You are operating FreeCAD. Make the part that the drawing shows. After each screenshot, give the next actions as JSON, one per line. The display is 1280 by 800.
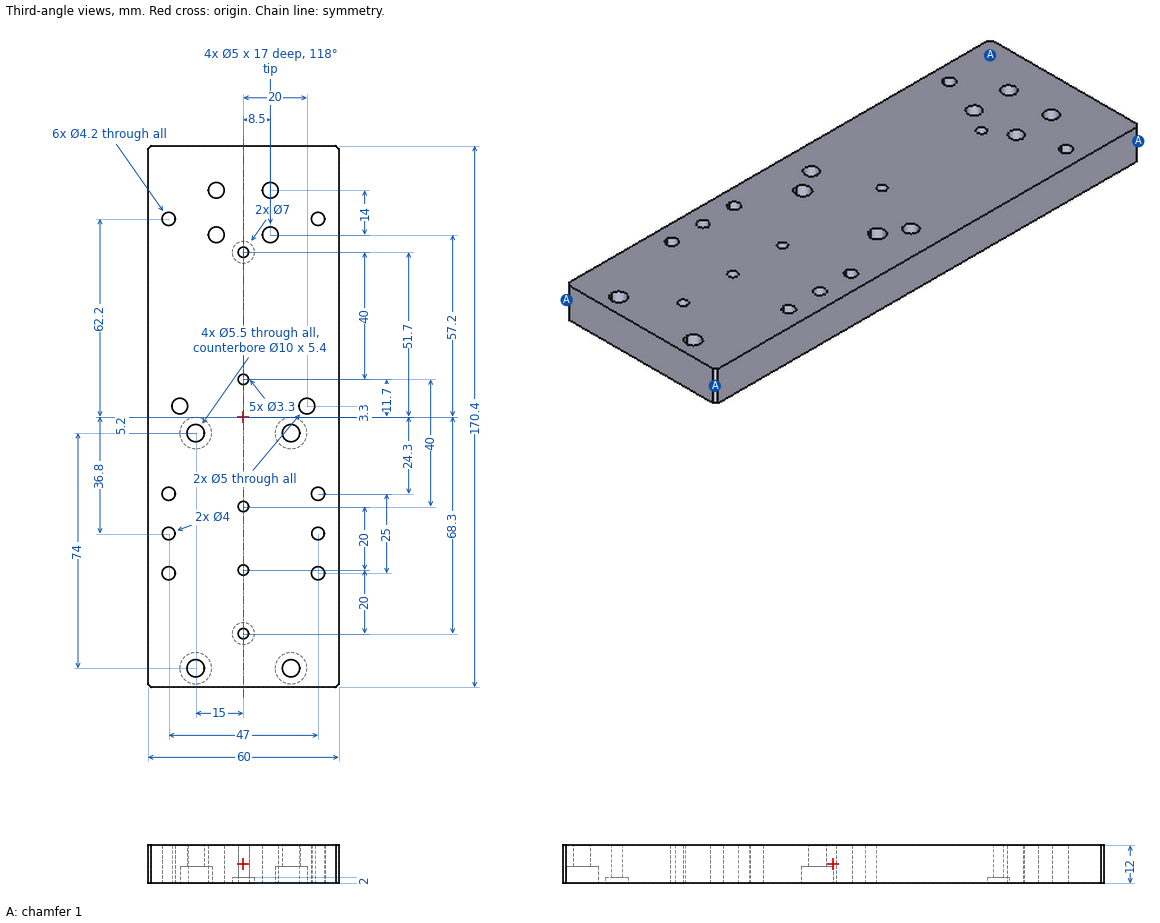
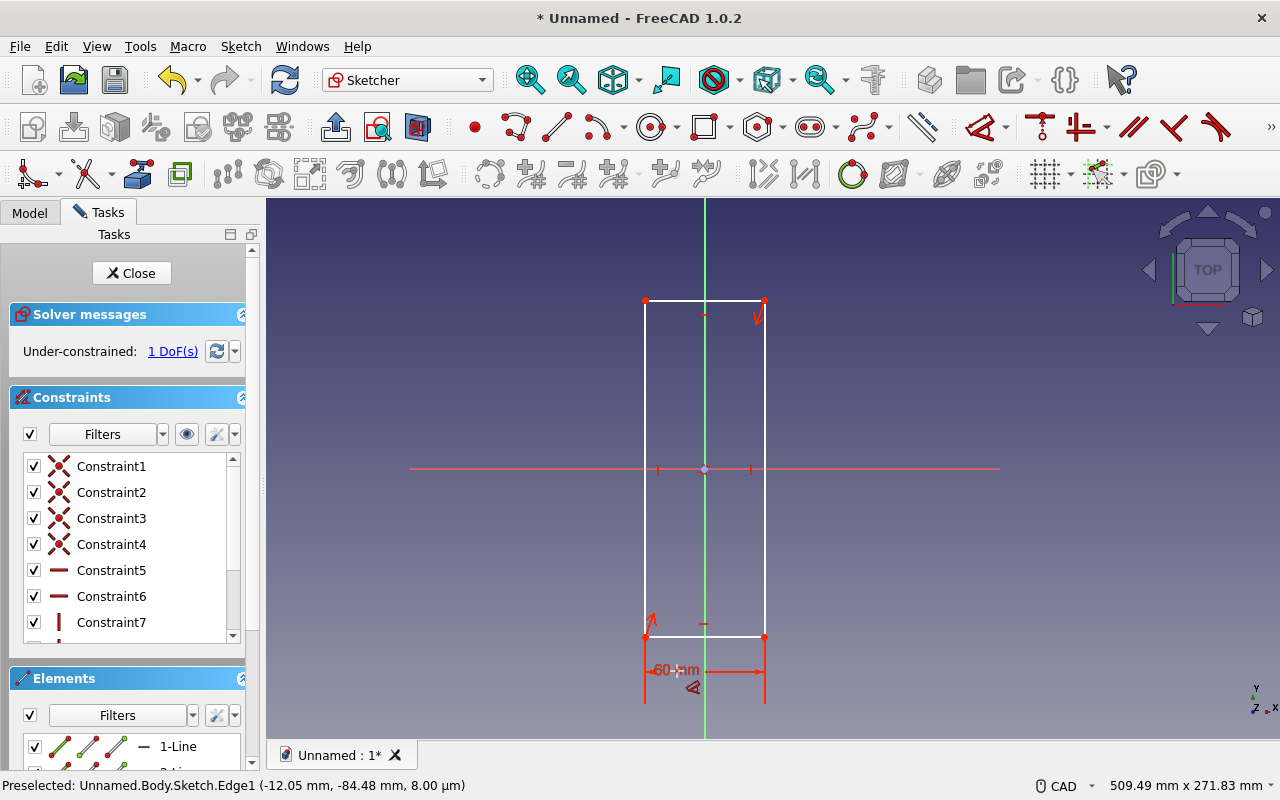
{"action": "left_click", "coordinate": [765, 536]}
{"action": "left_click", "coordinate": [799, 392]}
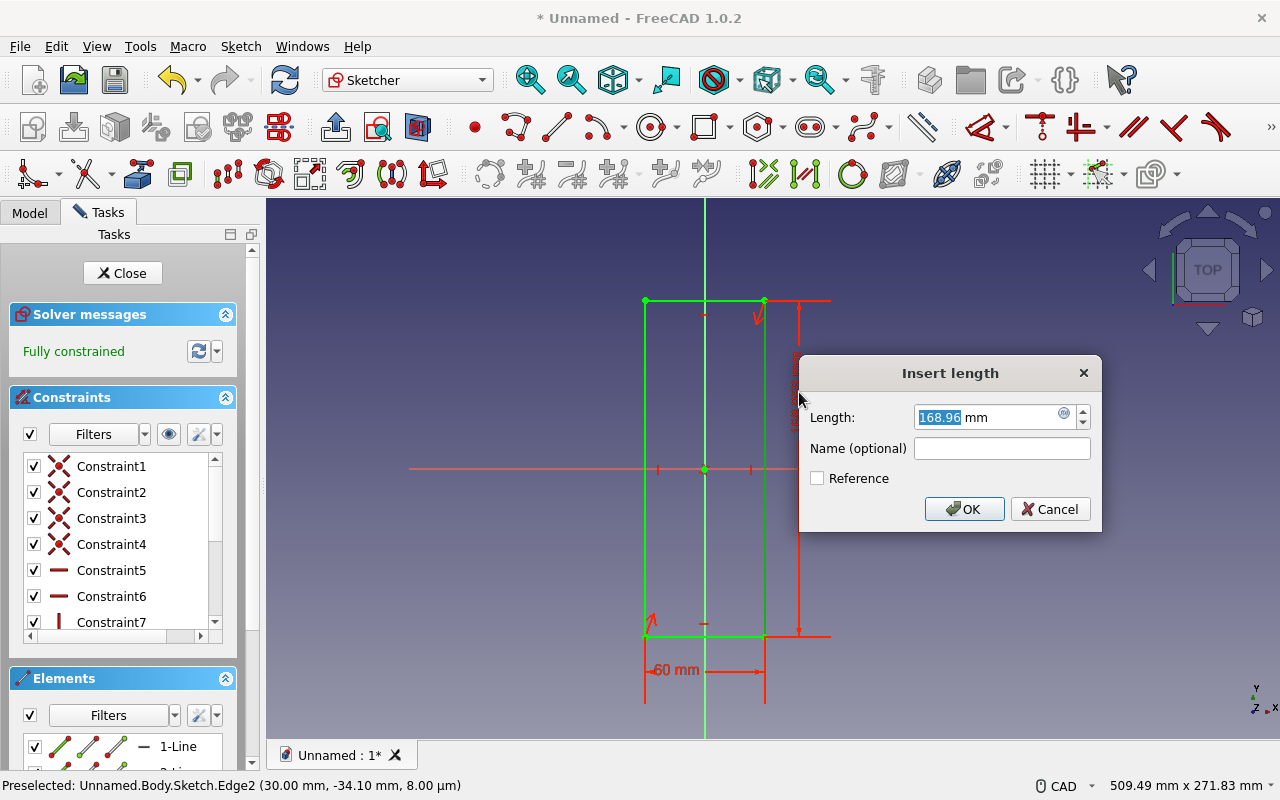
{"action": "type", "text": "170.4"}
{"action": "key", "text": "Return"}
{"action": "key", "text": "Escape"}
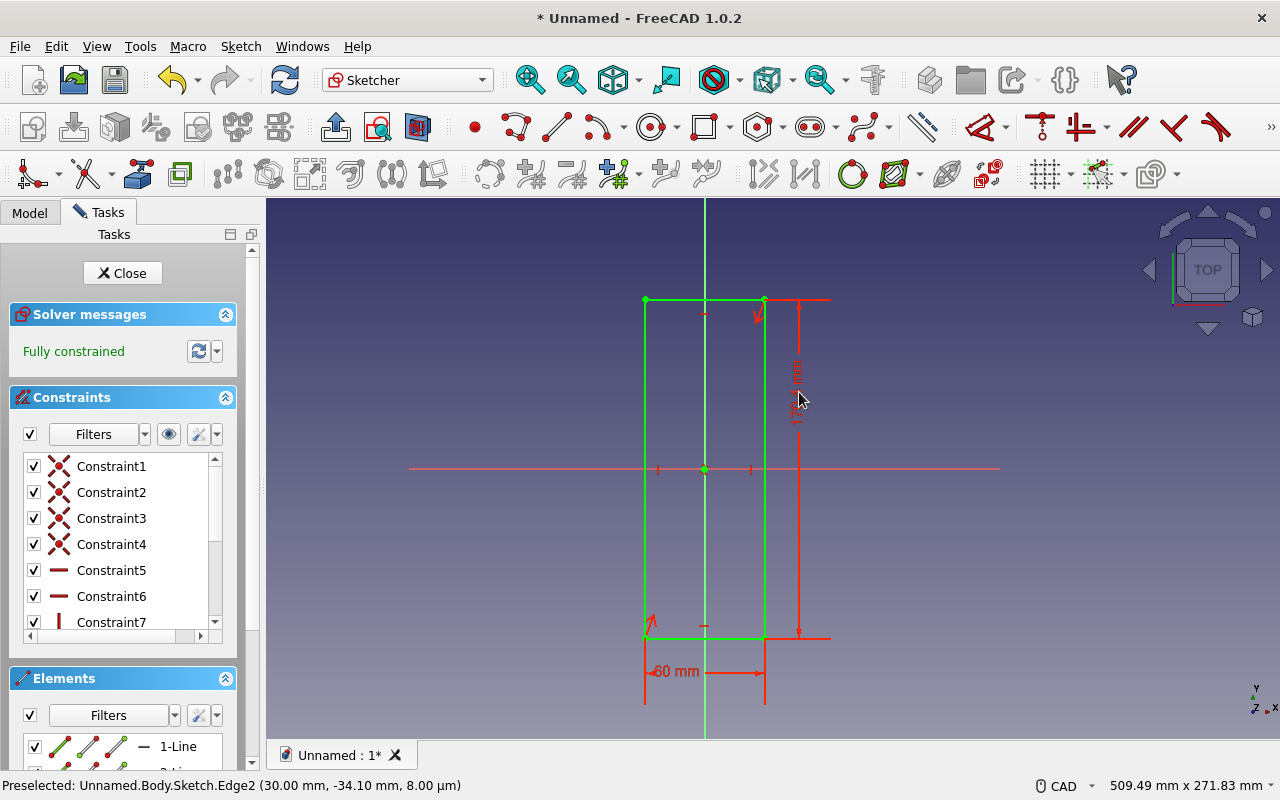
{"action": "left_click", "coordinate": [123, 273]}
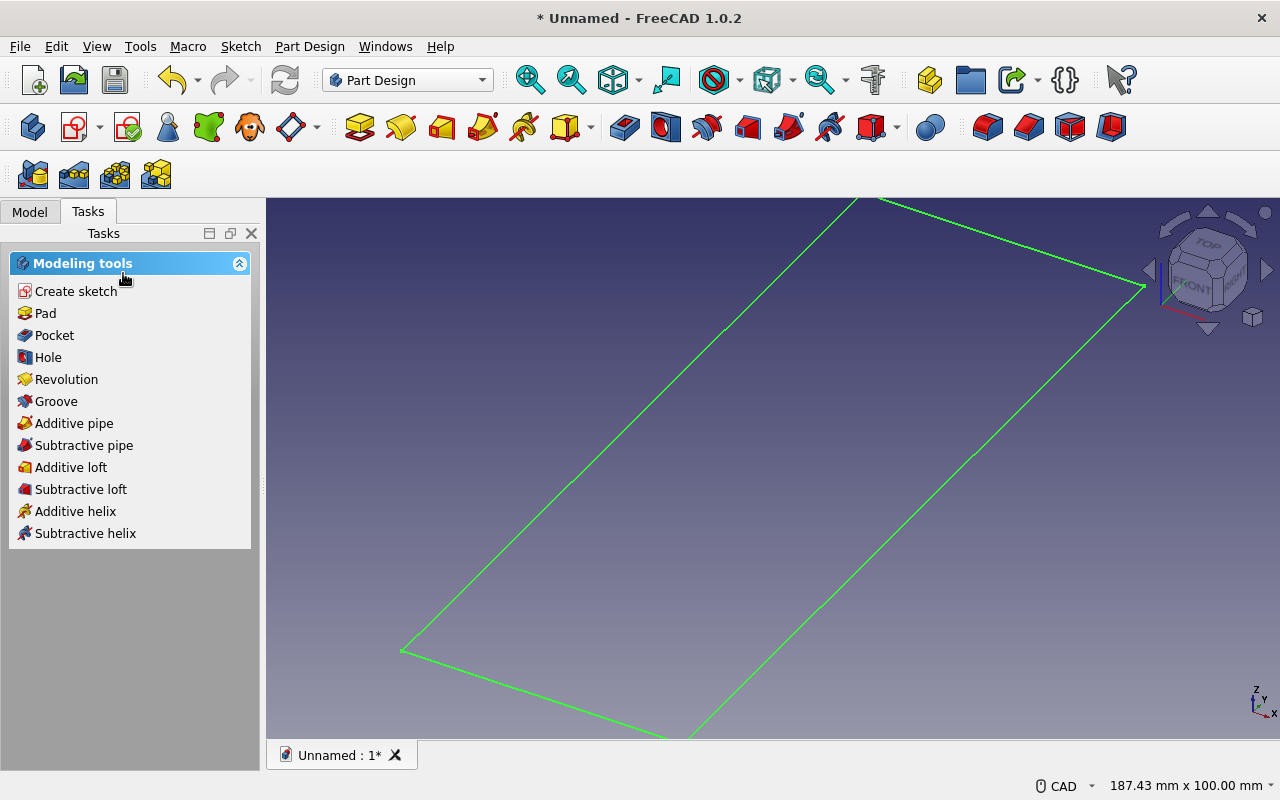
{"action": "left_click", "coordinate": [360, 128]}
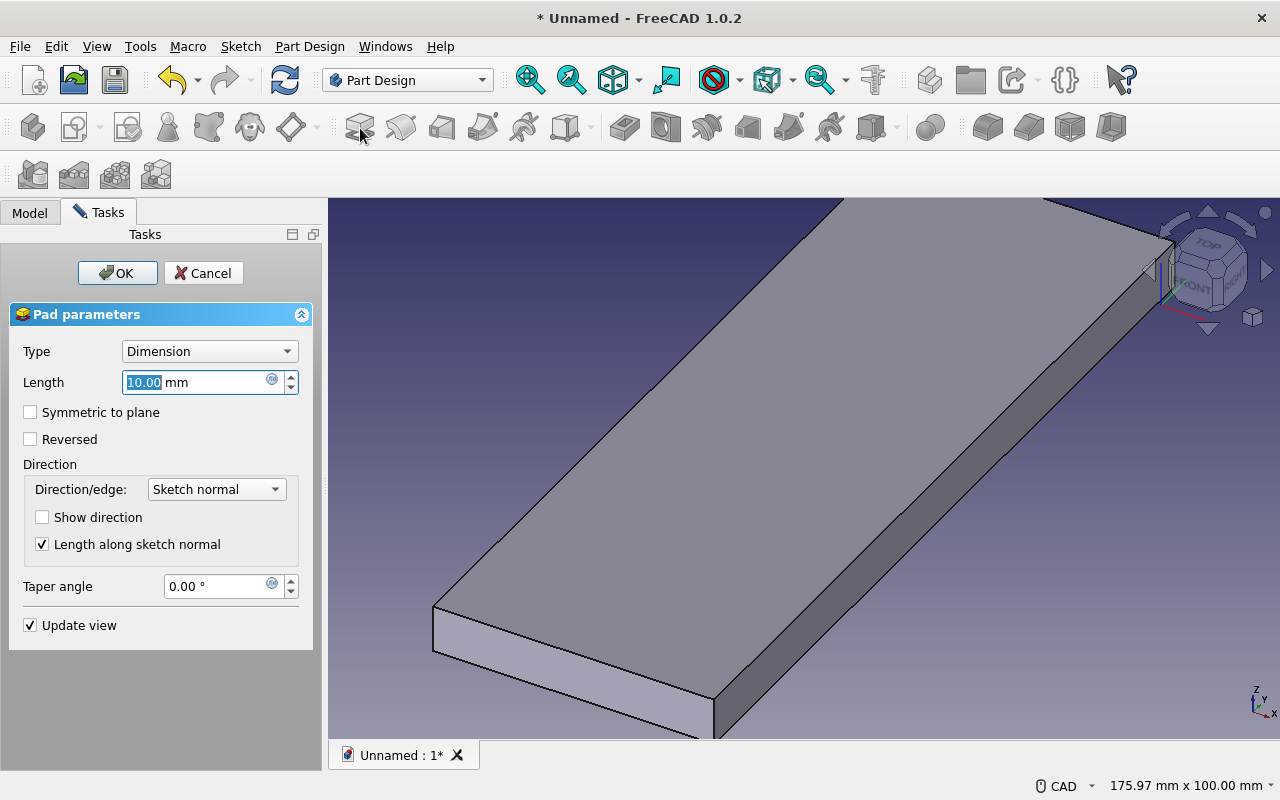
{"action": "type", "text": "12"}
{"action": "key", "text": "Tab"}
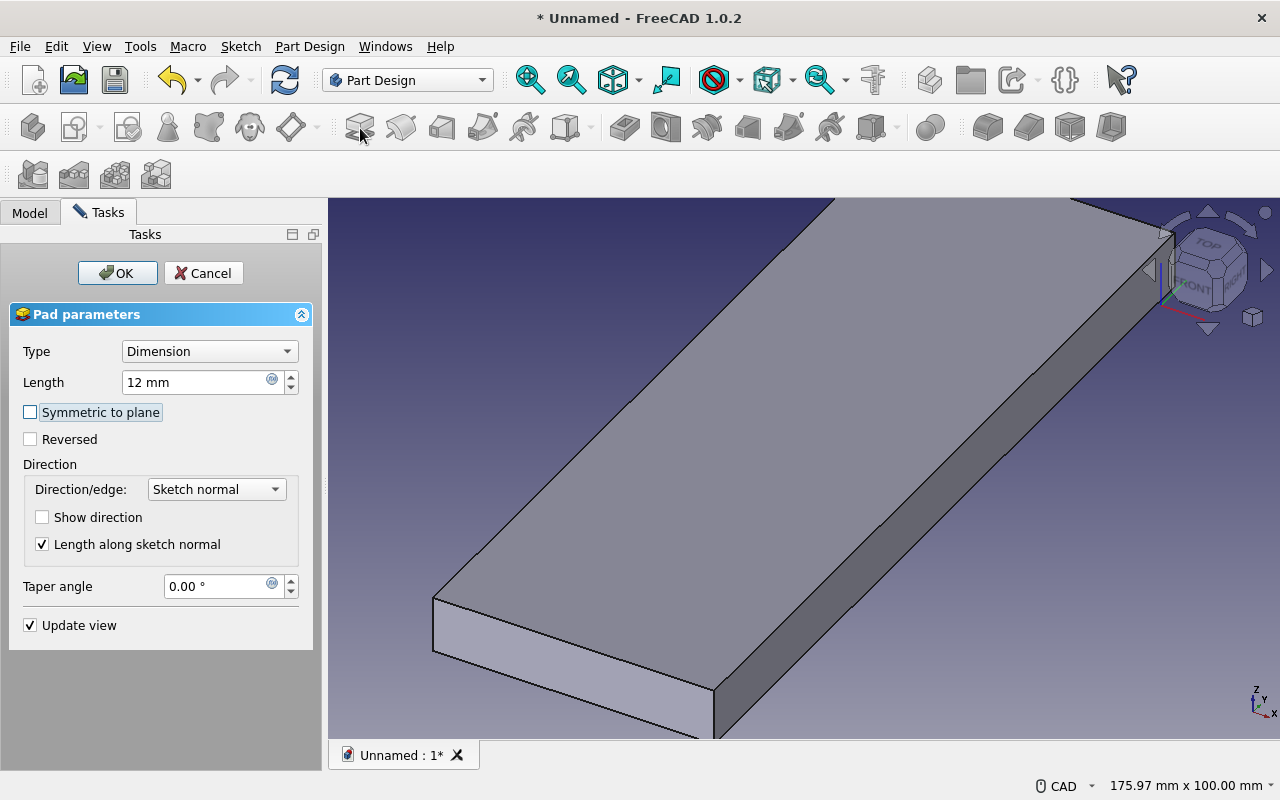
{"action": "left_click", "coordinate": [31, 412]}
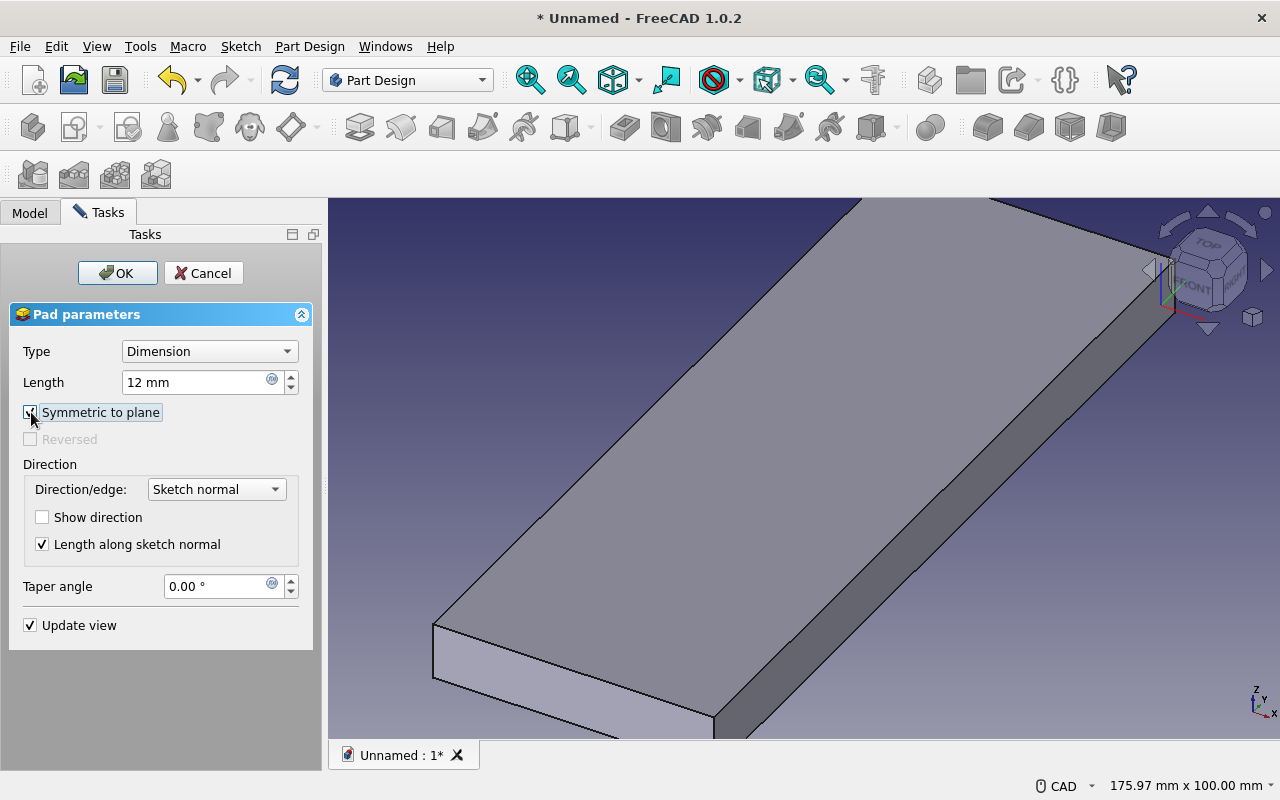
{"action": "left_click", "coordinate": [118, 273]}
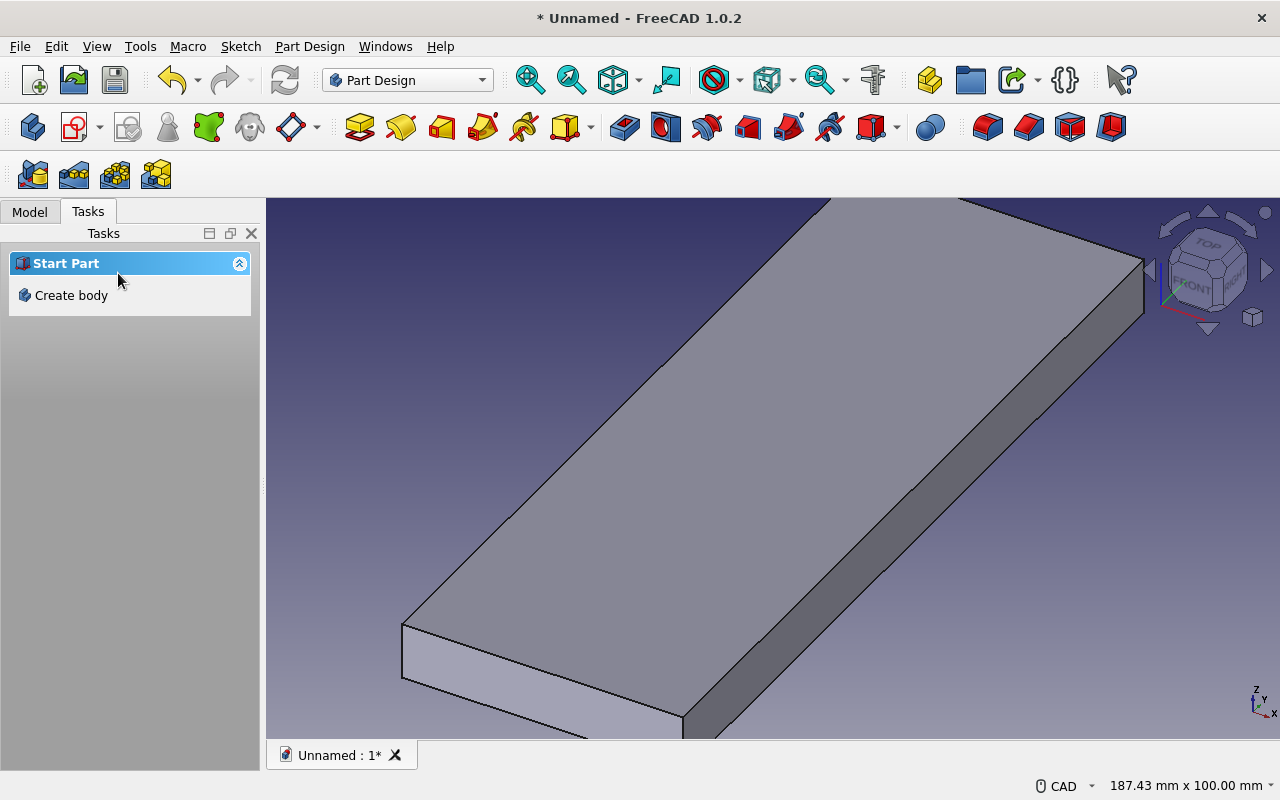
{"action": "left_click", "coordinate": [531, 80]}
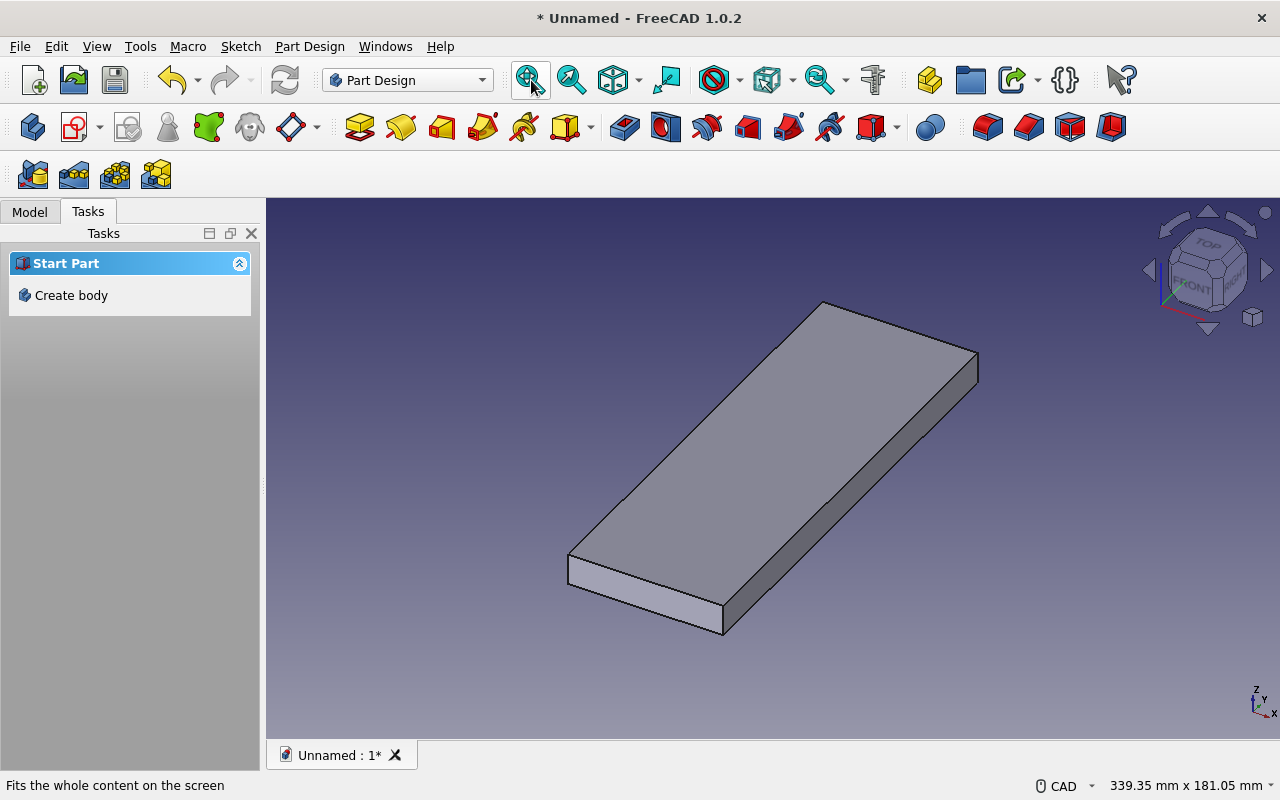
{"action": "key", "text": "5"}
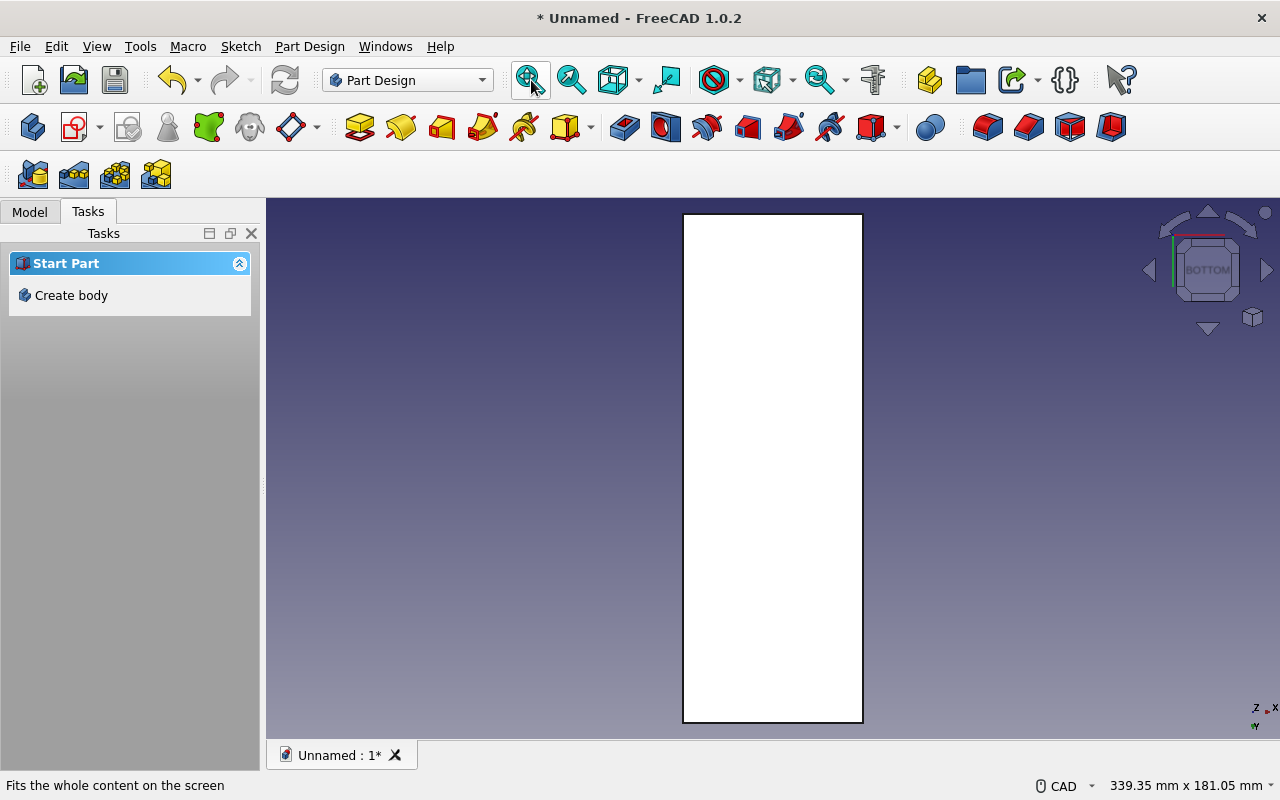
{"action": "left_click", "coordinate": [773, 613]}